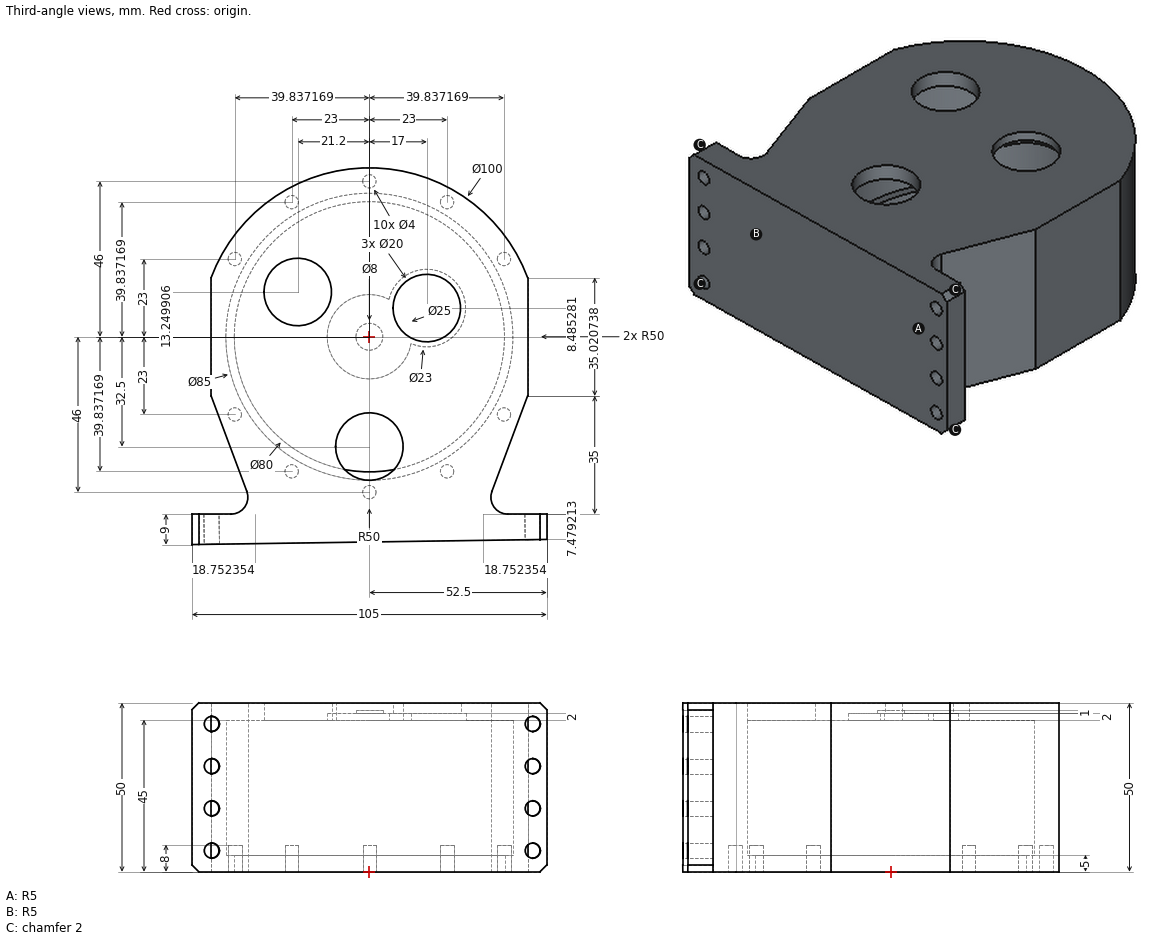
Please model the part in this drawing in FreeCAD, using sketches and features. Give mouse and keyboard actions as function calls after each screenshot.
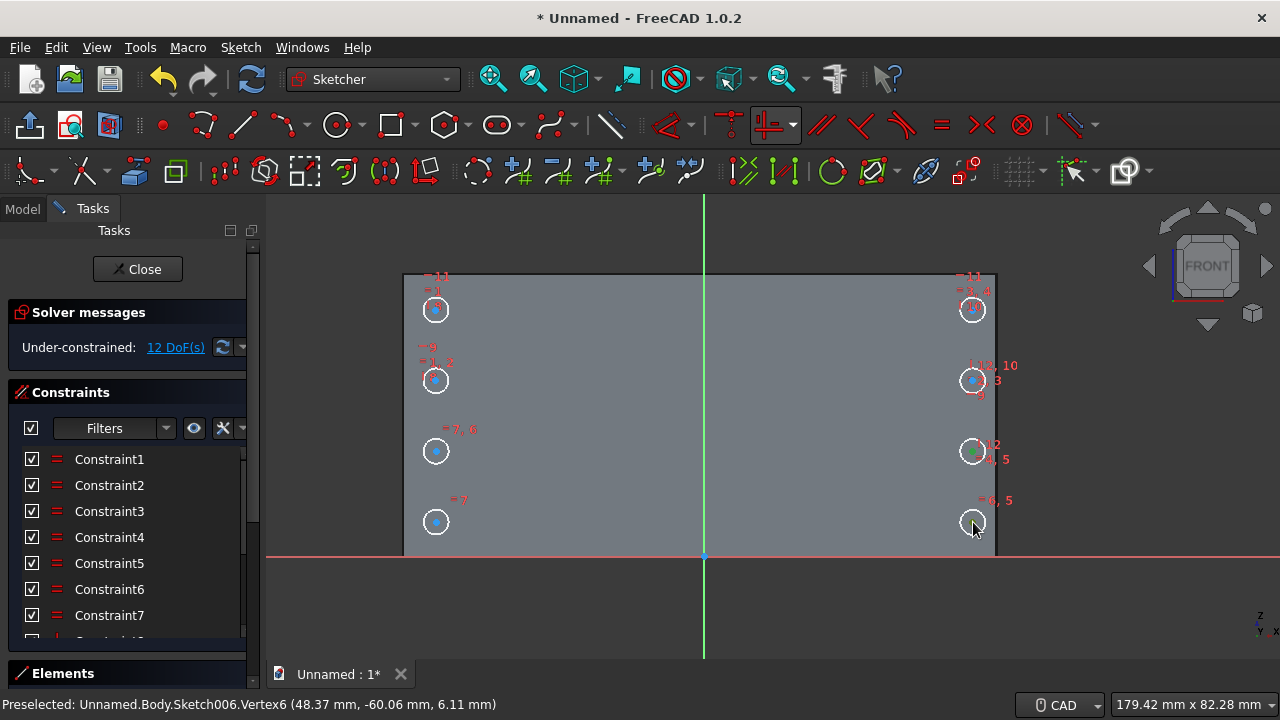
click(796, 126)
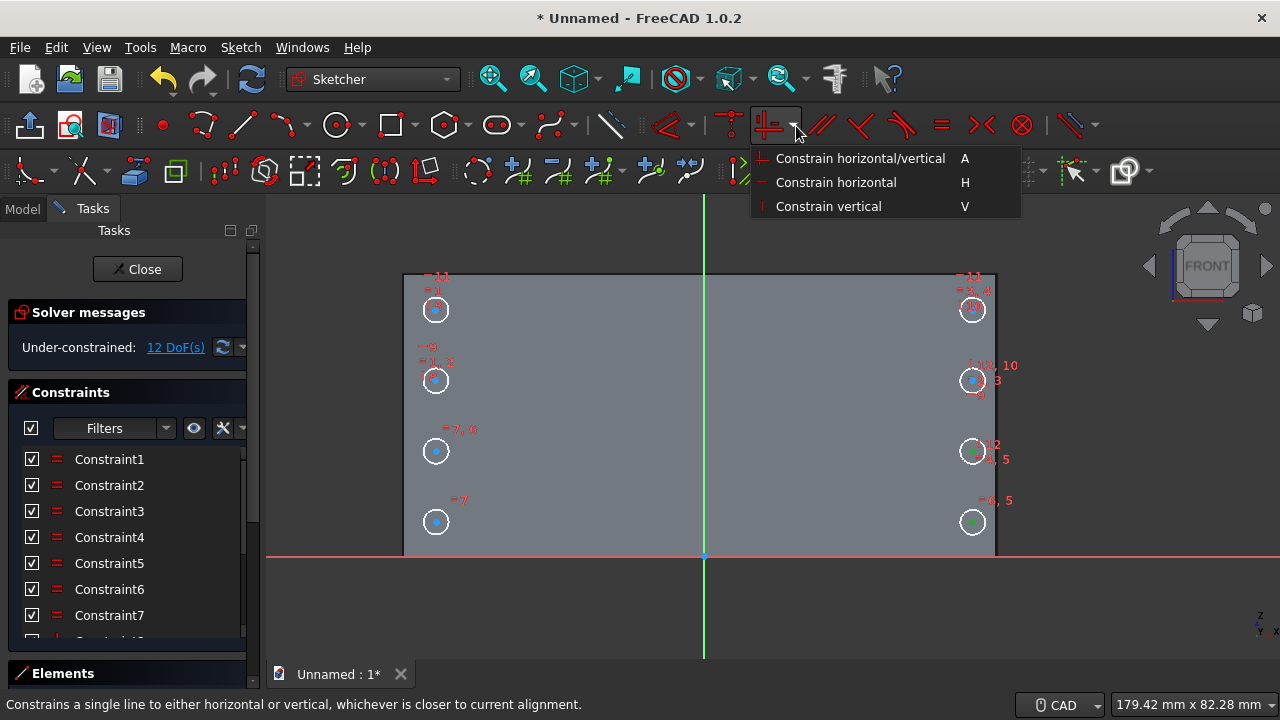
click(886, 206)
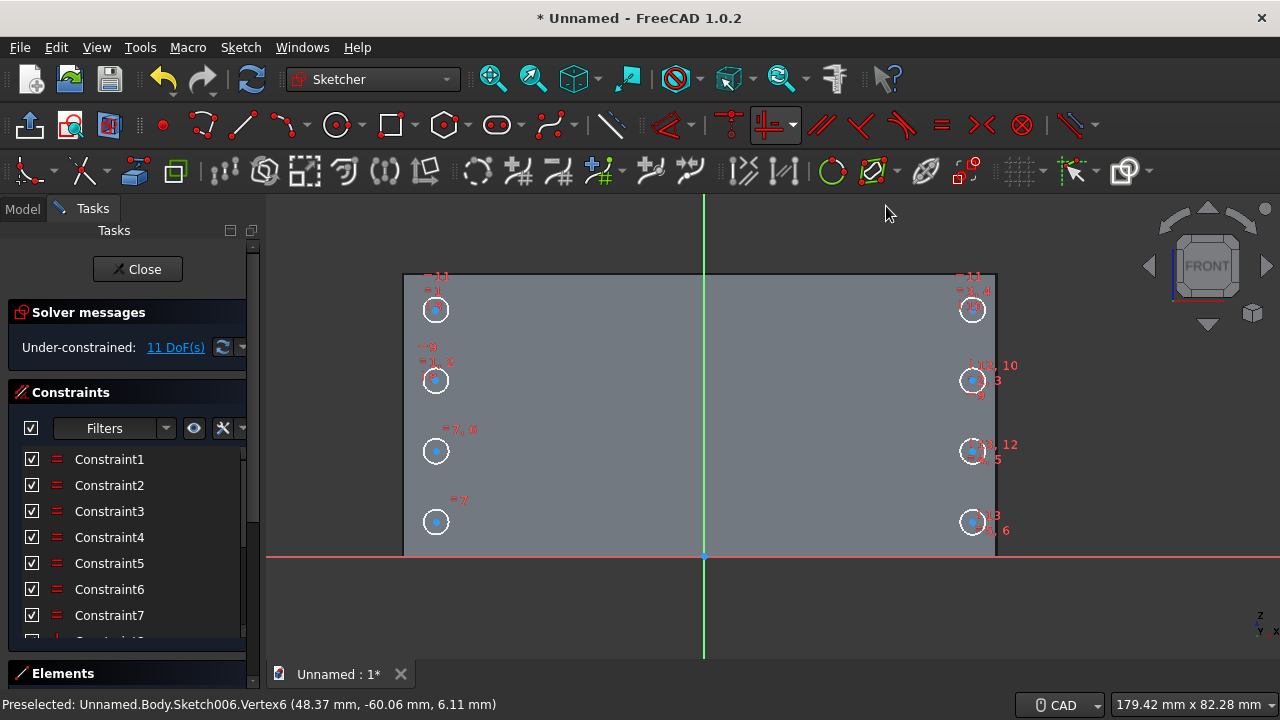
click(436, 381)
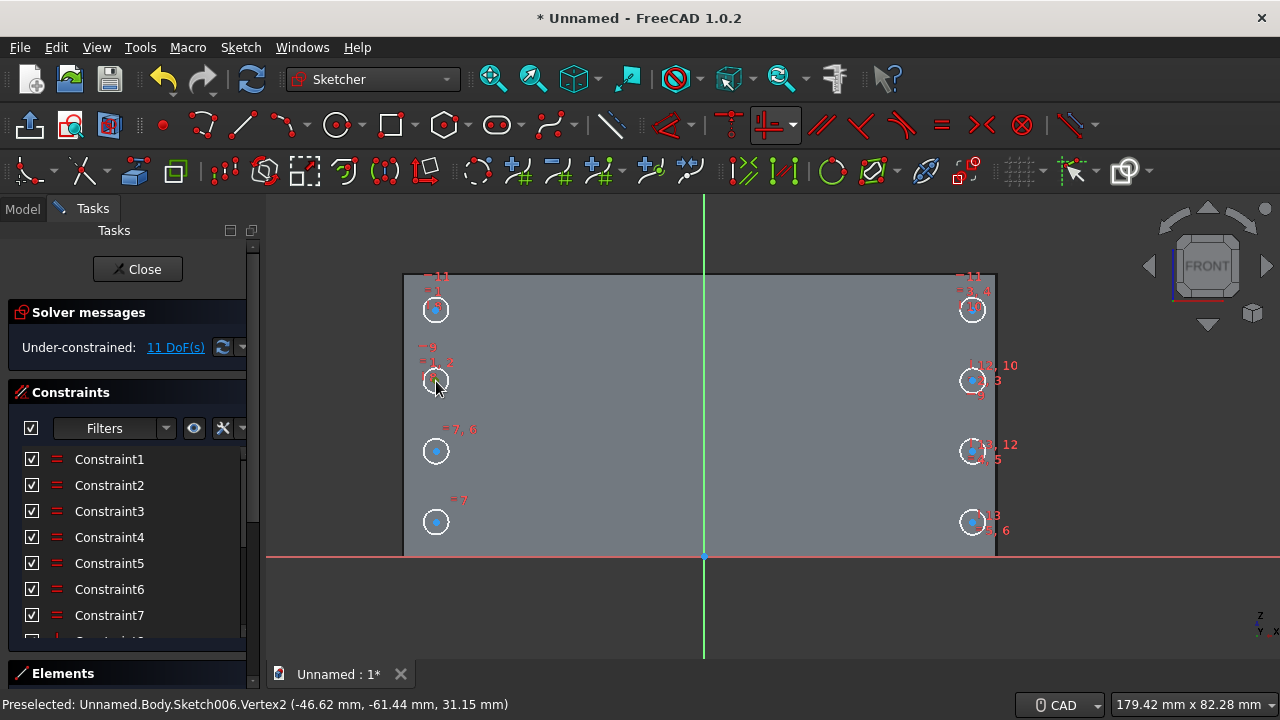
click(436, 451)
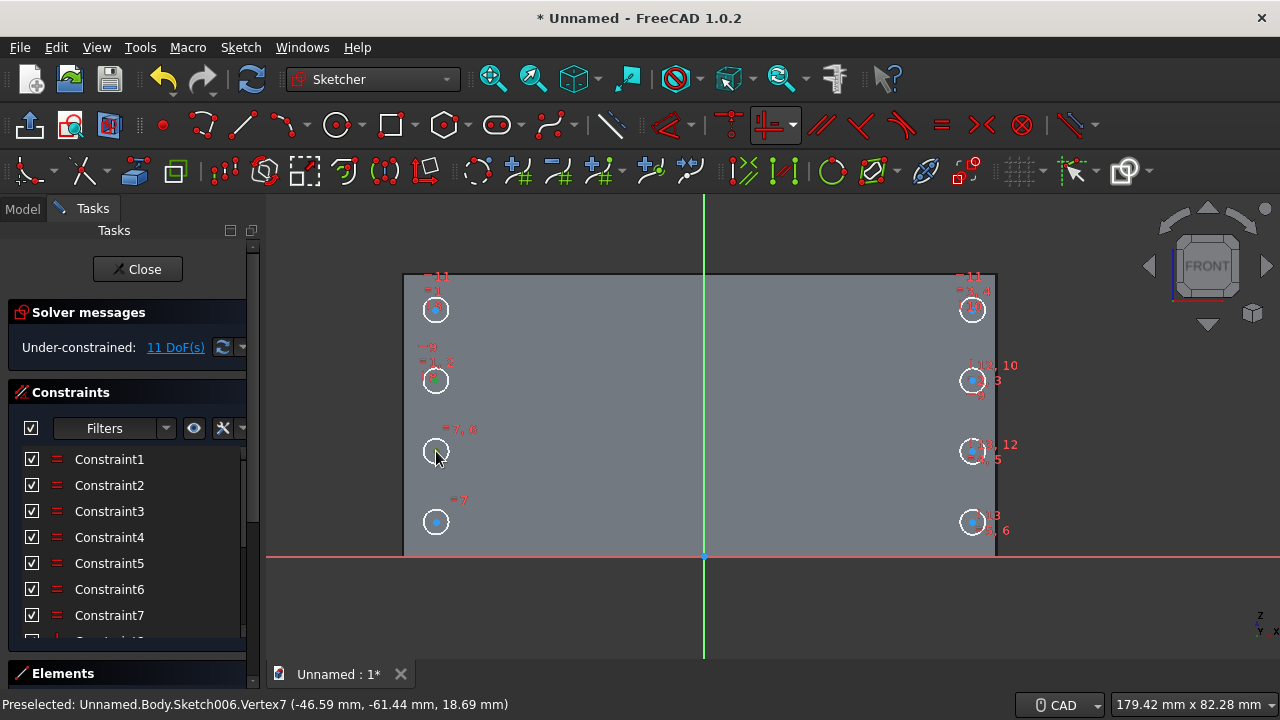
click(796, 126)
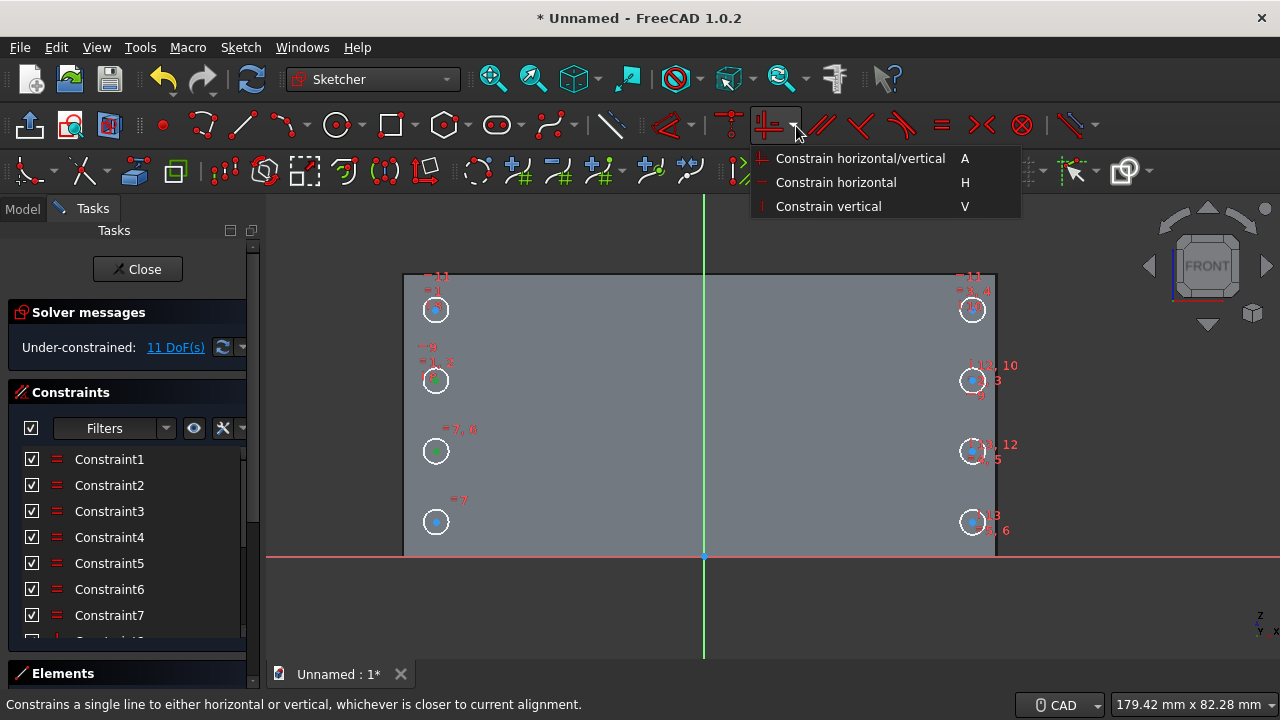
click(886, 206)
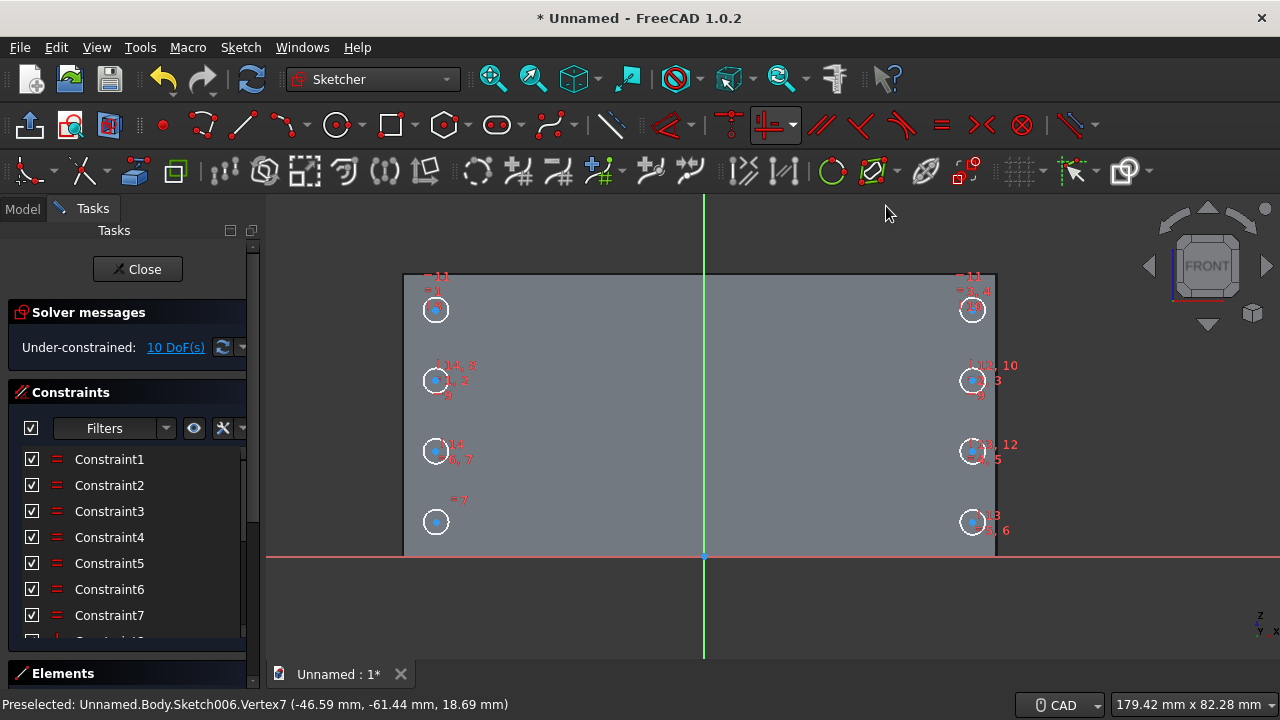
click(973, 451)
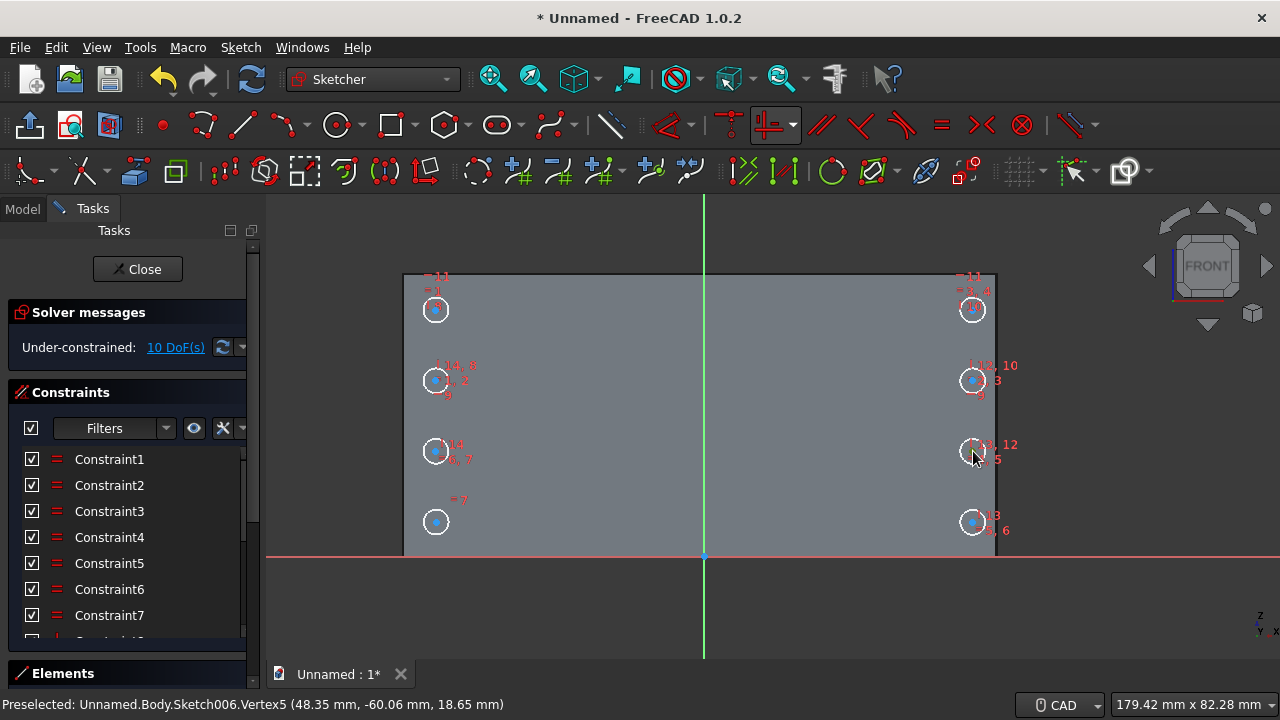
click(436, 451)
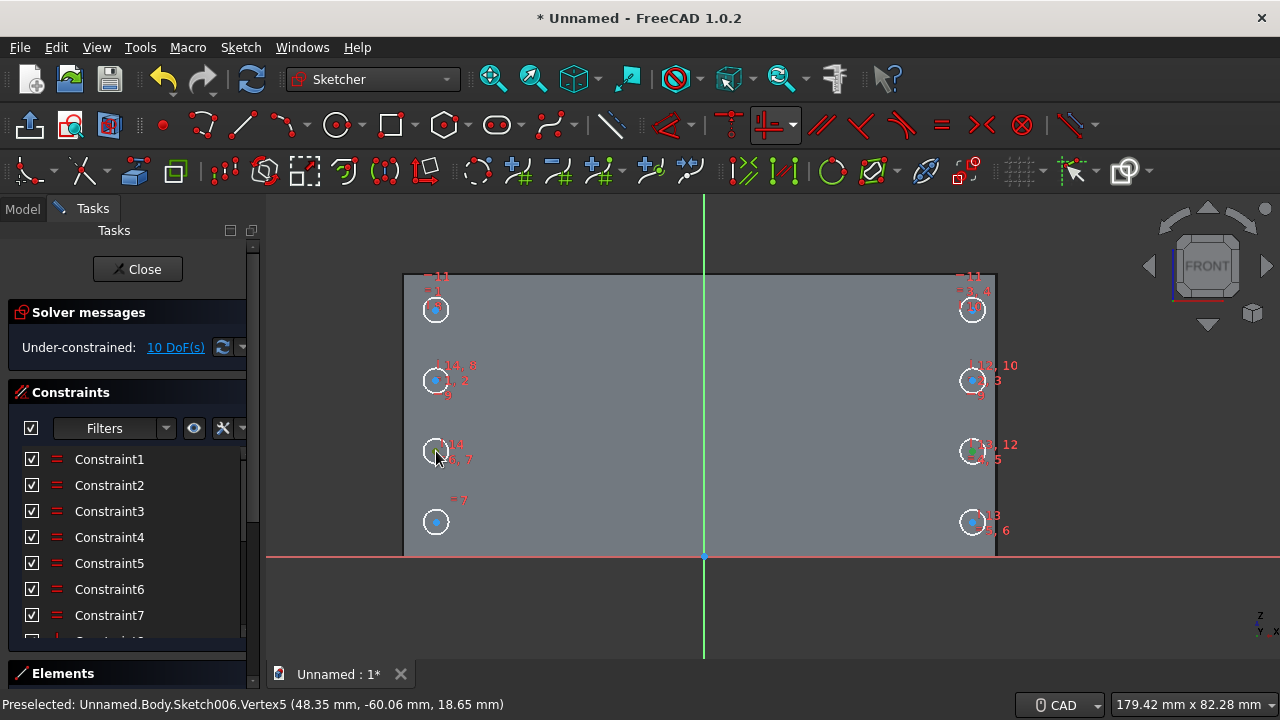
key(h)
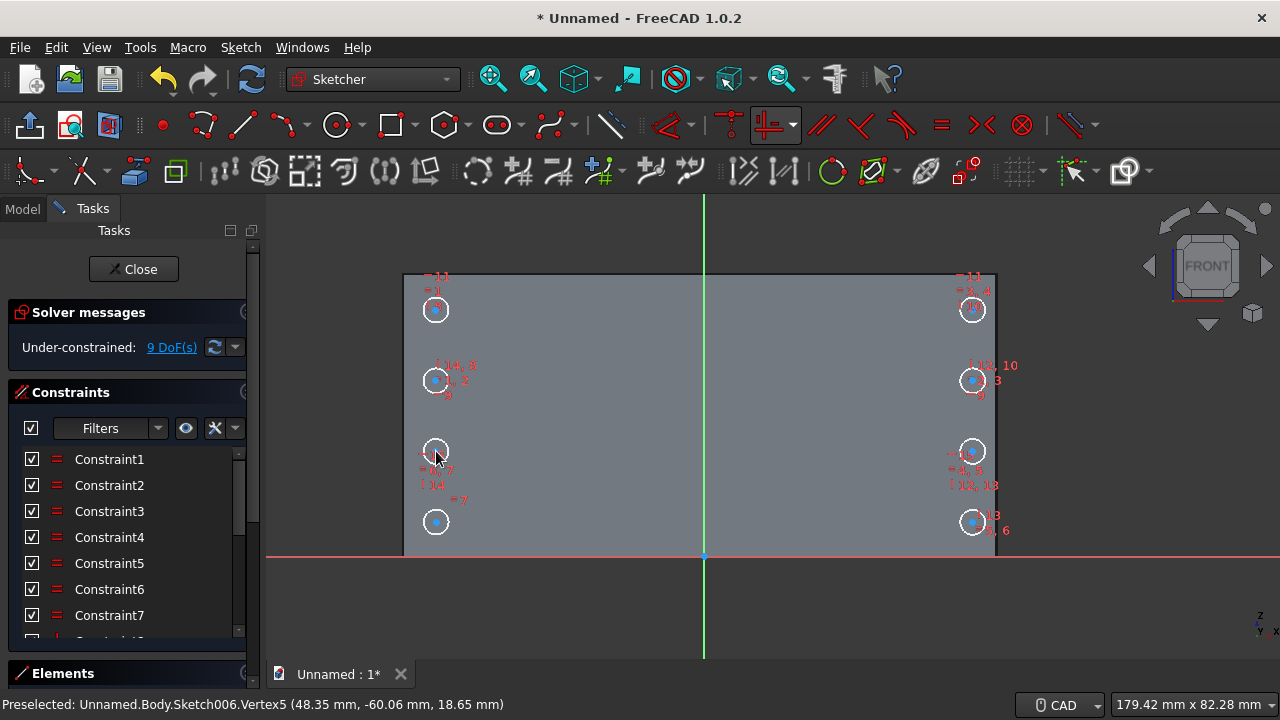
scroll(436, 451, up, 4)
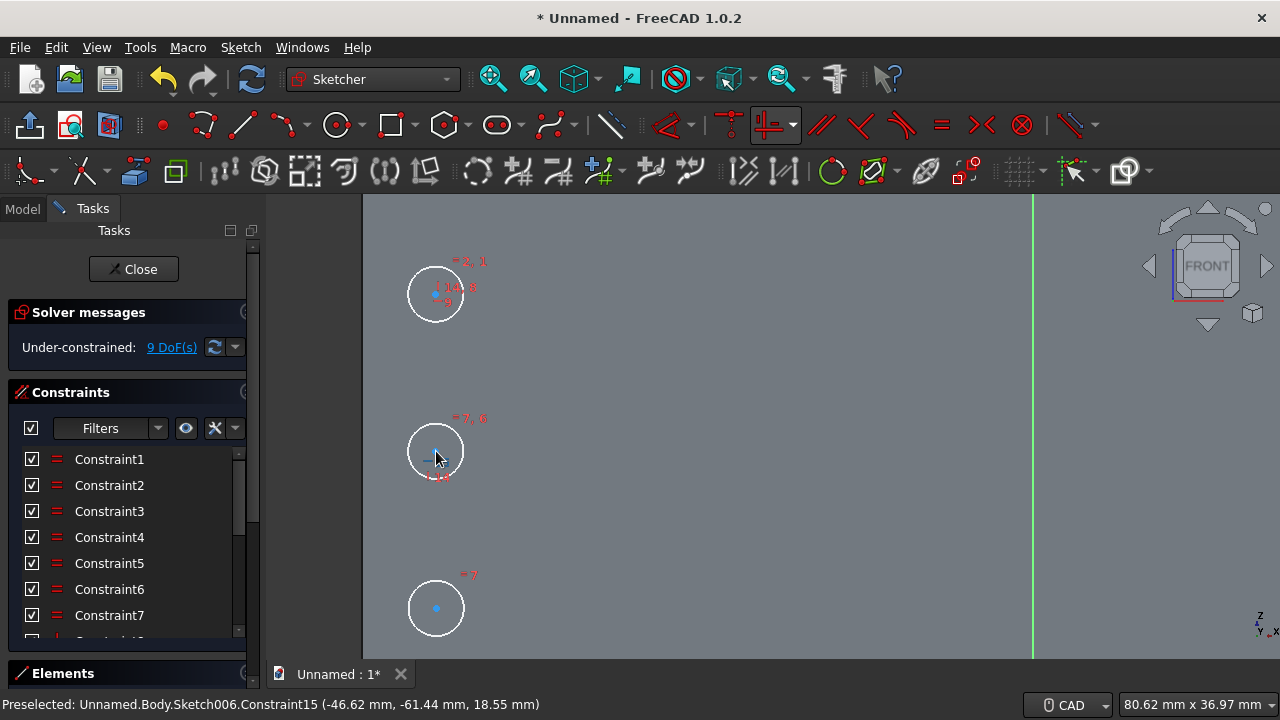
click(436, 451)